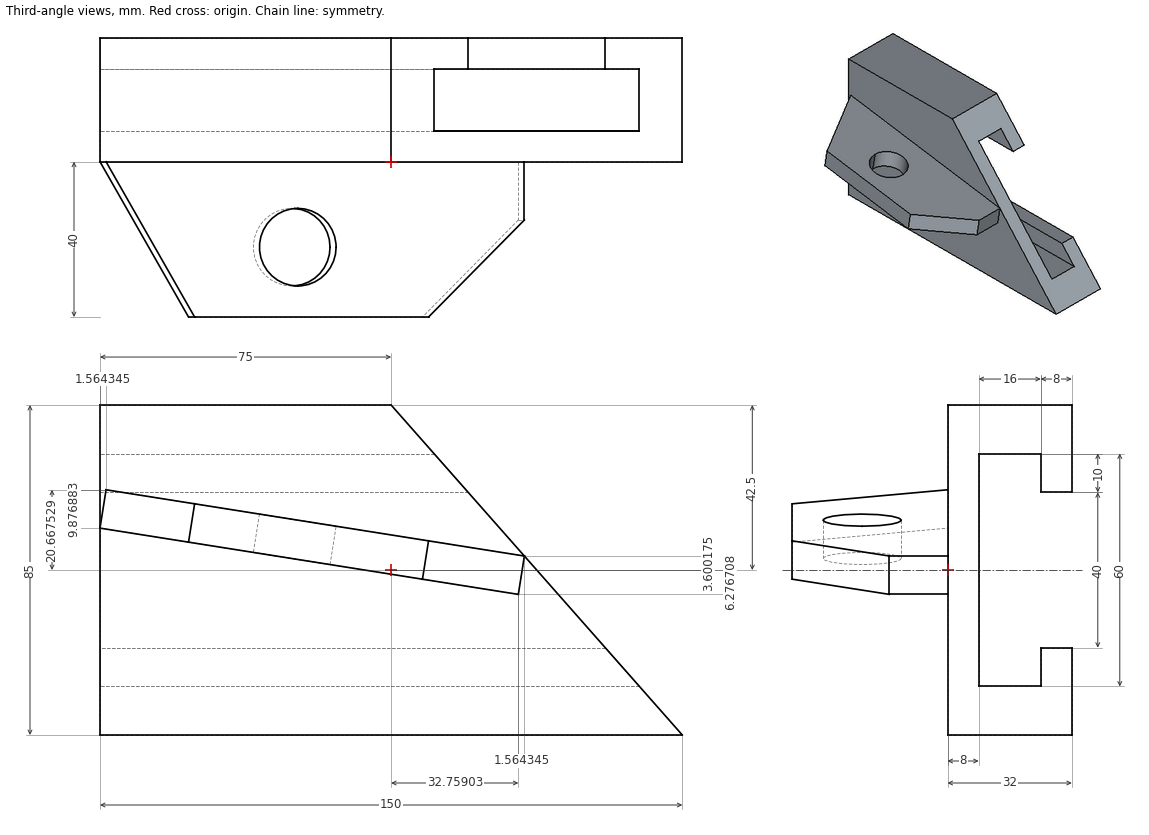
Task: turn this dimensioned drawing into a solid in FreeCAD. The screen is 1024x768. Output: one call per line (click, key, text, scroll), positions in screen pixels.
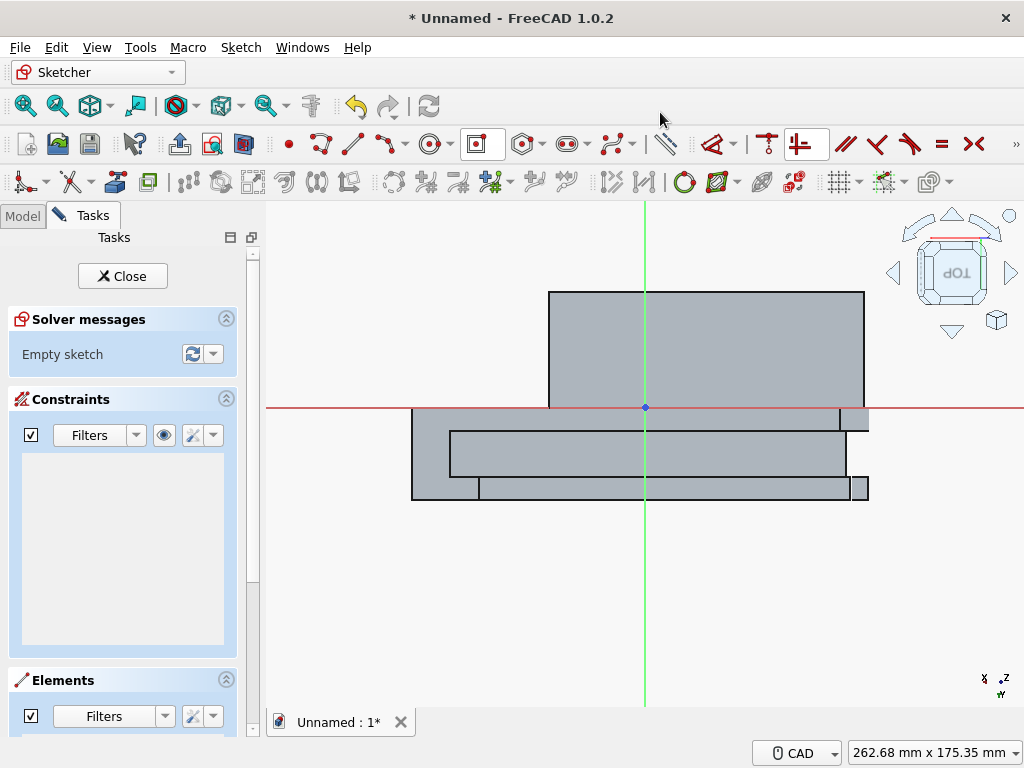
scroll(294, 679, down, 1)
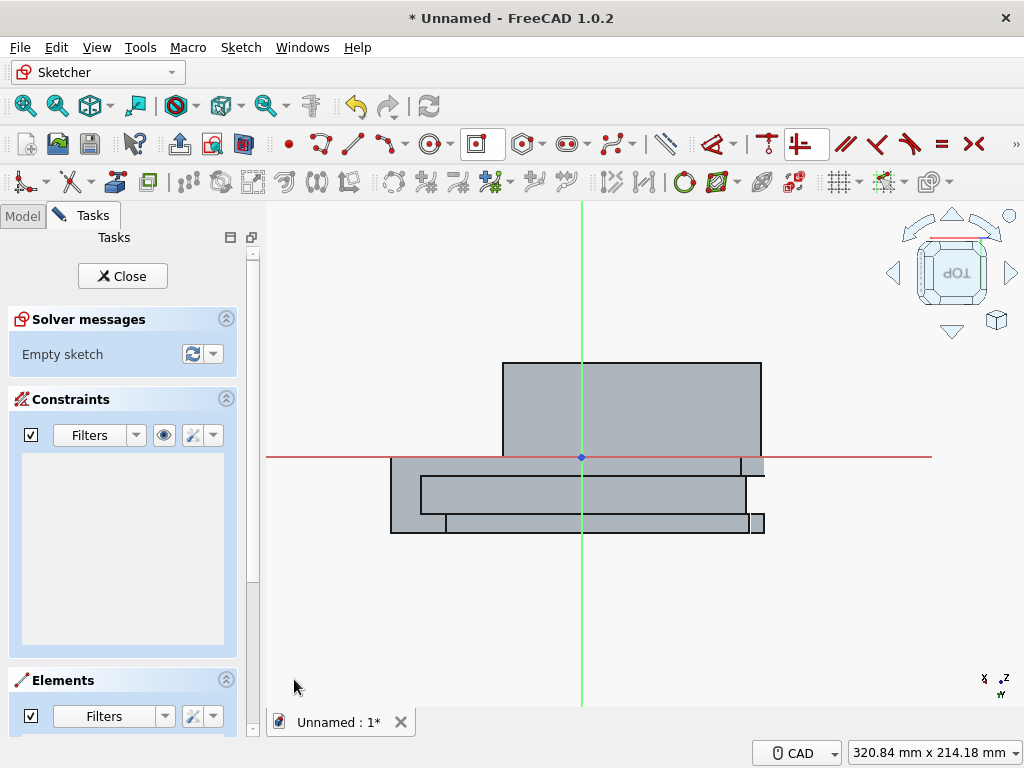
scroll(744, 320, up, 2)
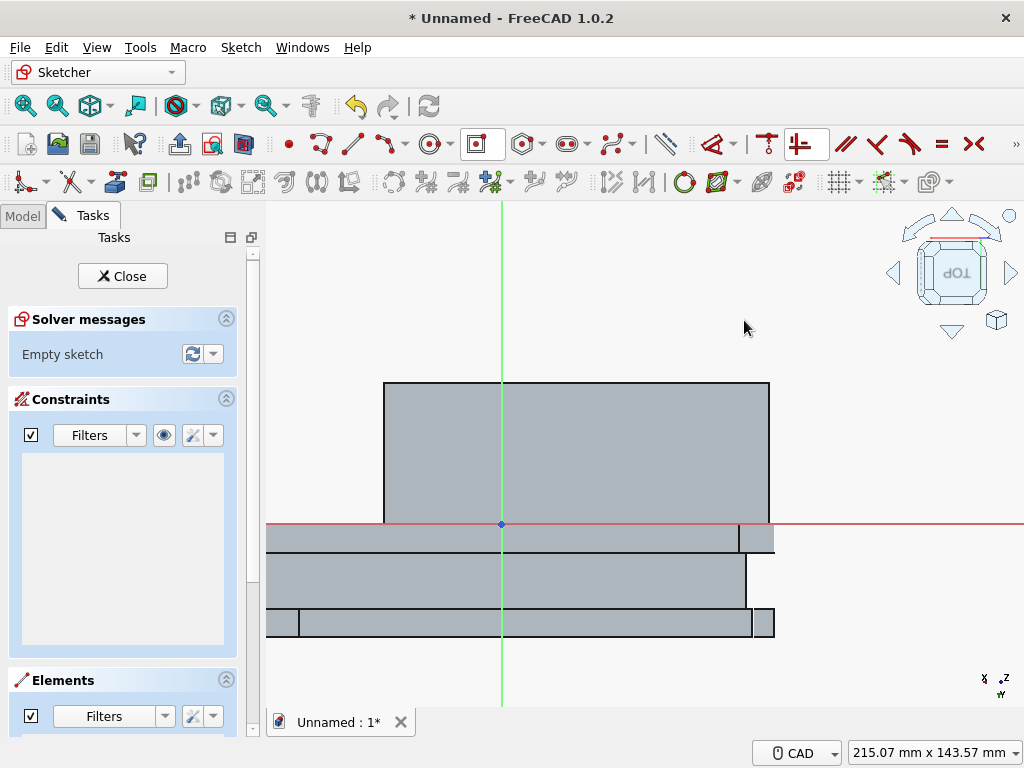
click(322, 144)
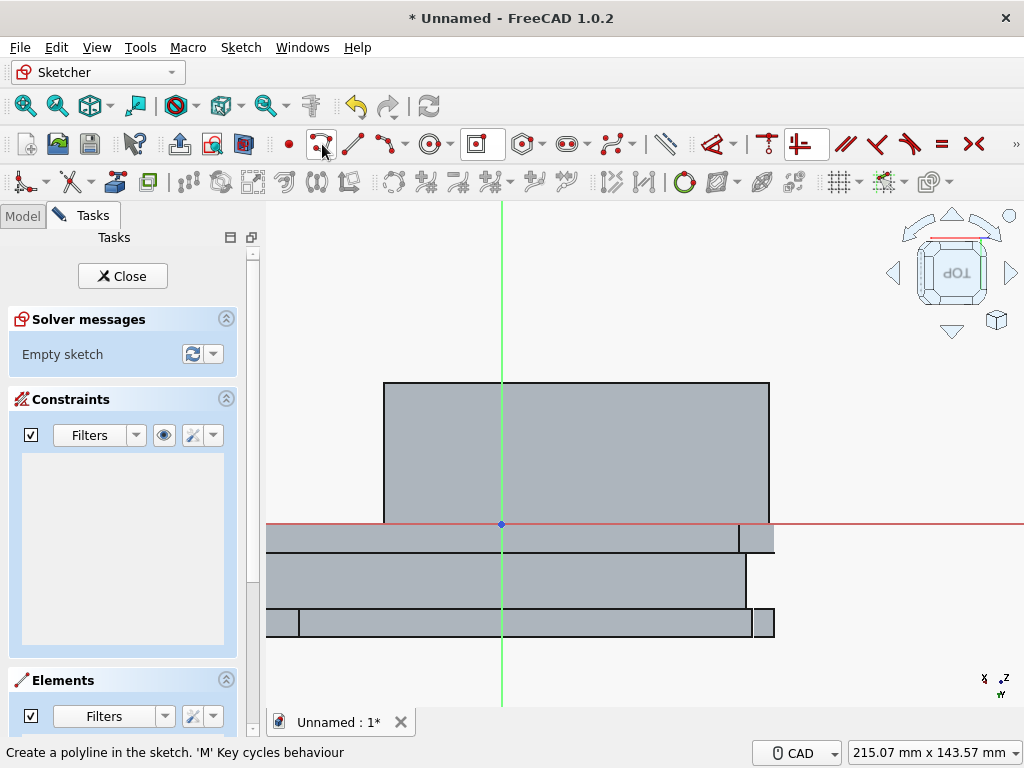
click(384, 471)
click(472, 383)
click(384, 383)
click(384, 472)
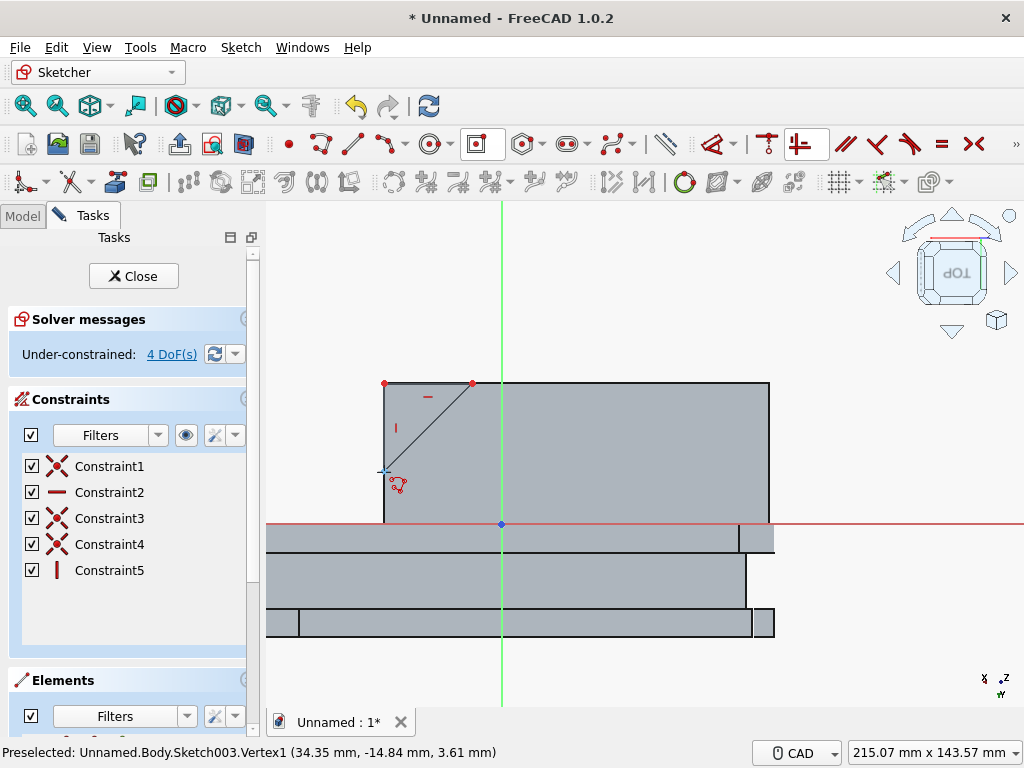
click(687, 383)
click(769, 524)
click(769, 383)
click(687, 384)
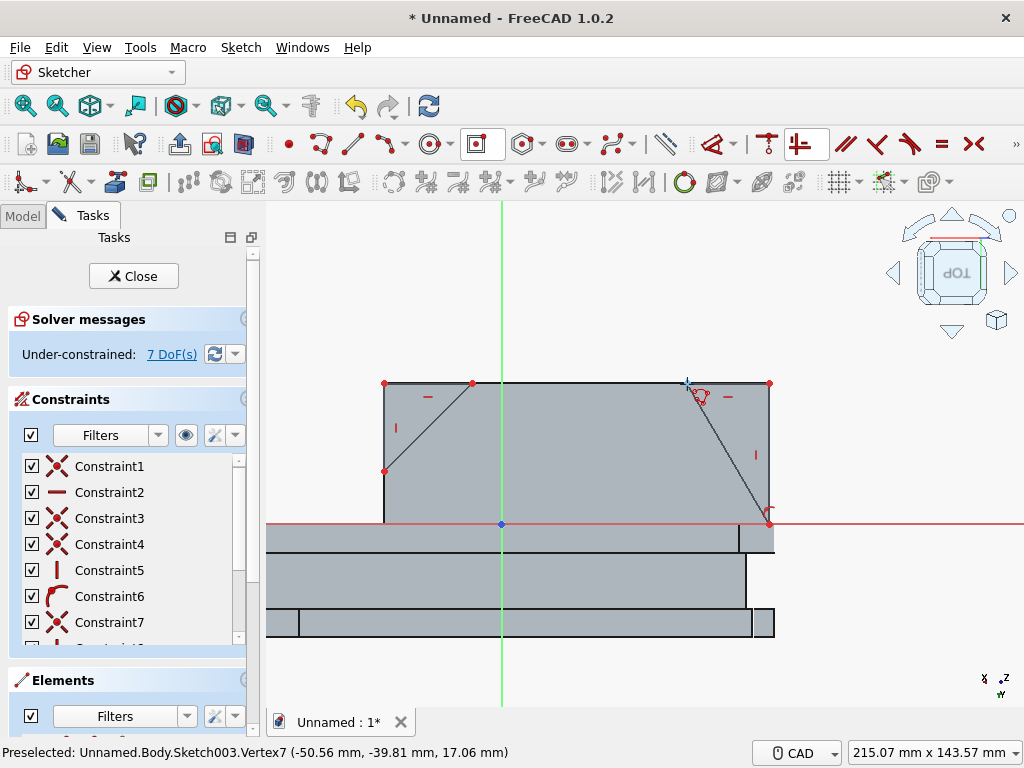
click(430, 144)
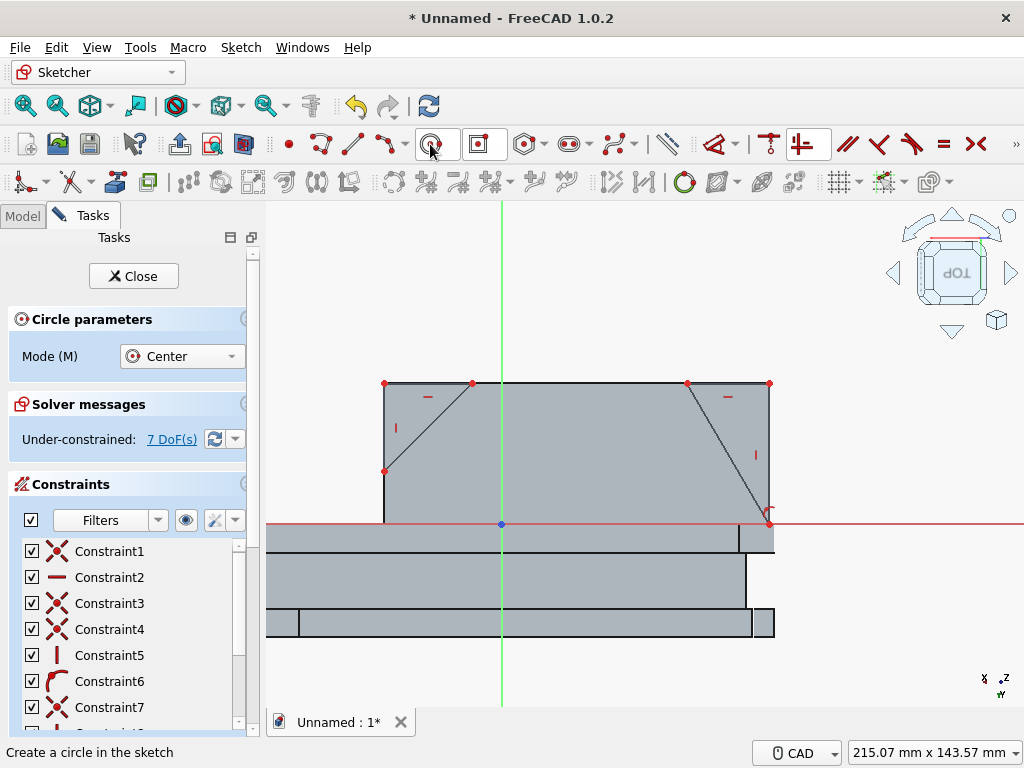
click(592, 447)
move(617, 422)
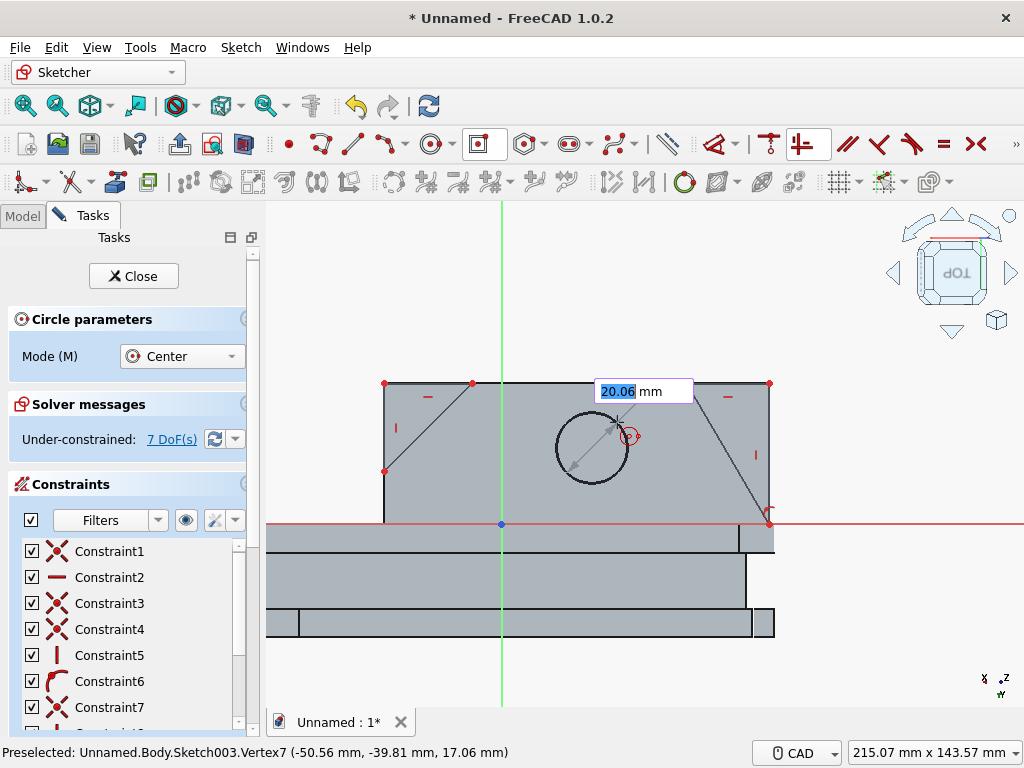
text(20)
key(Return)
key(Escape)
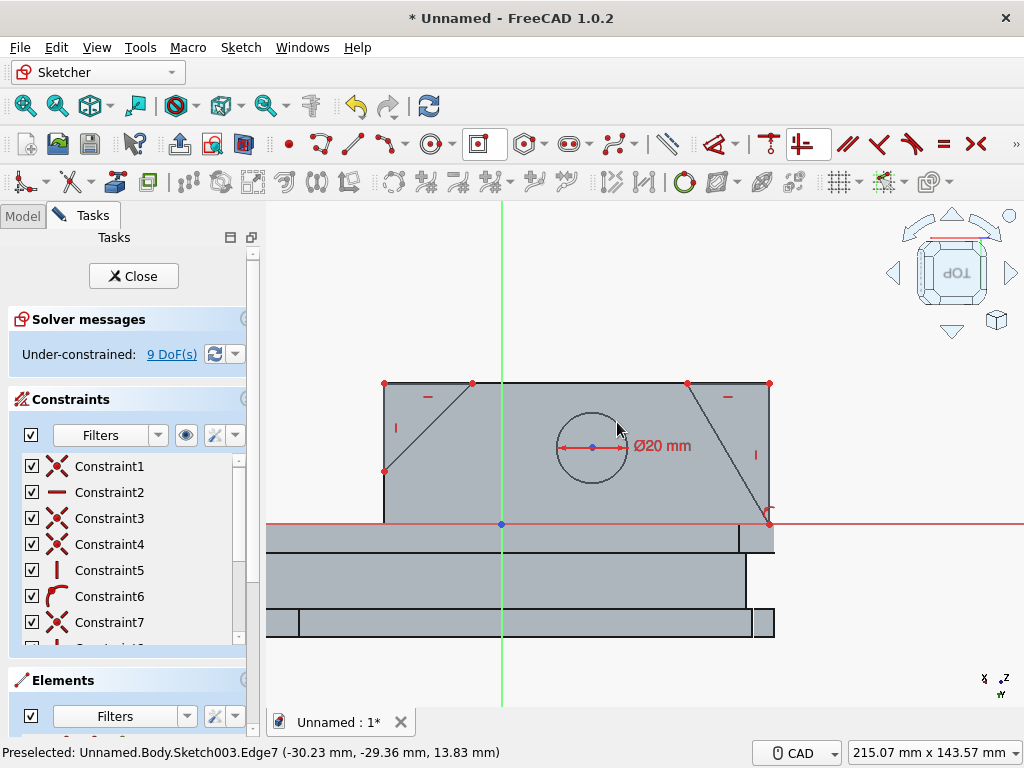
key(d)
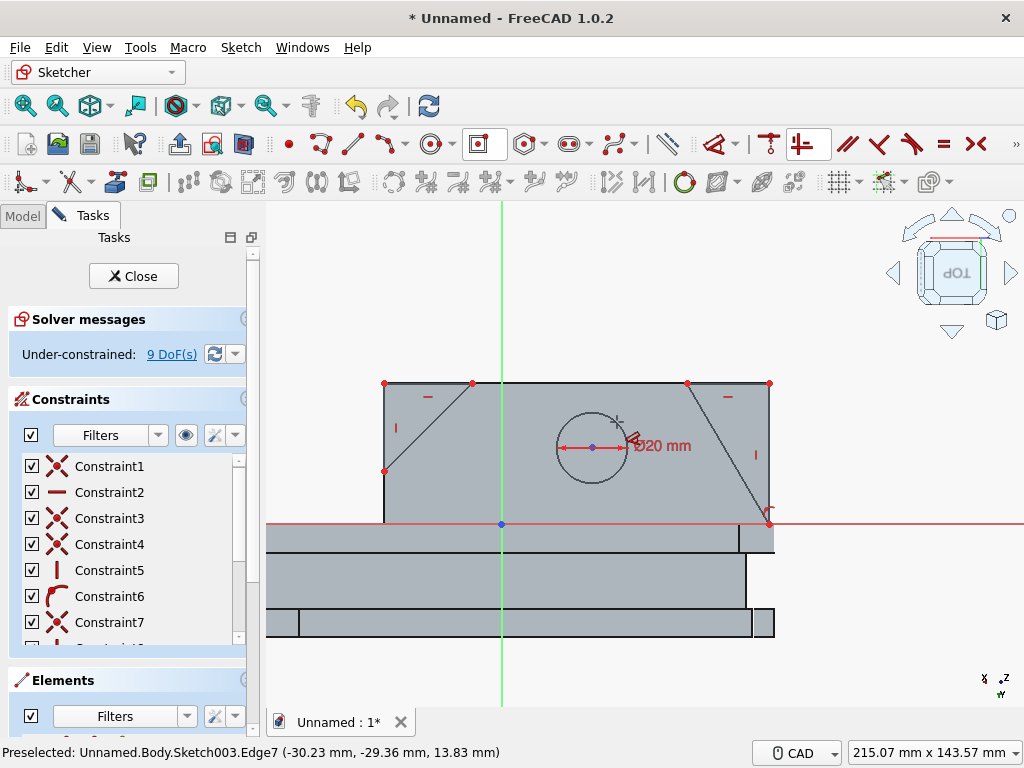
click(446, 384)
click(428, 350)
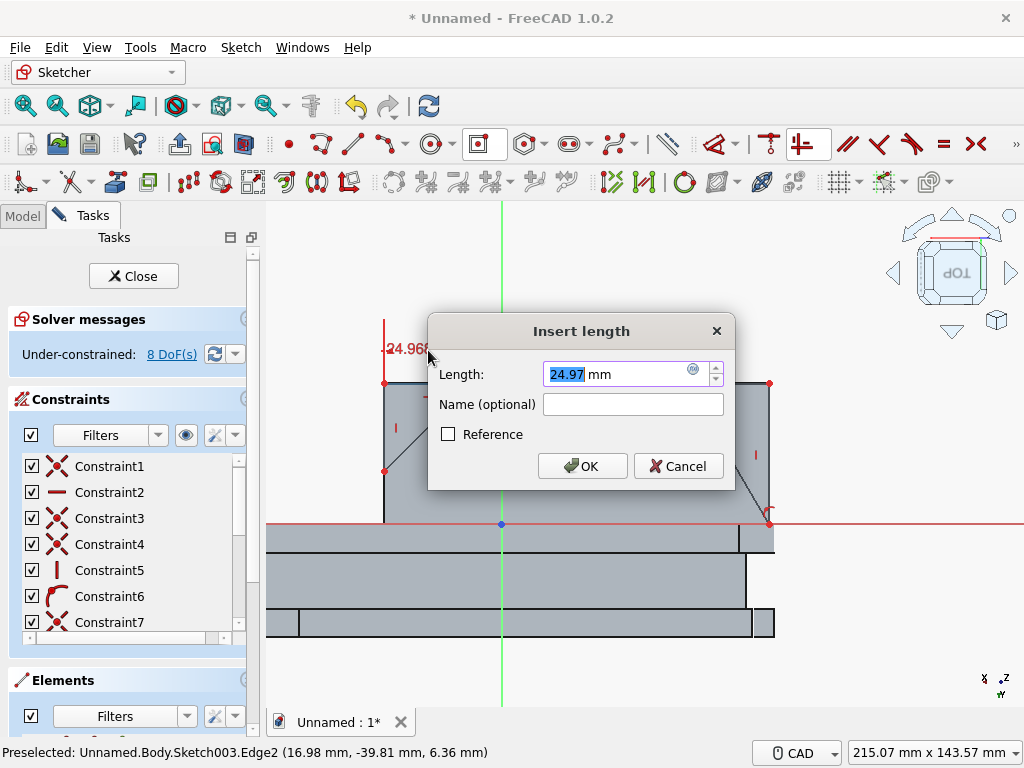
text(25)
key(Return)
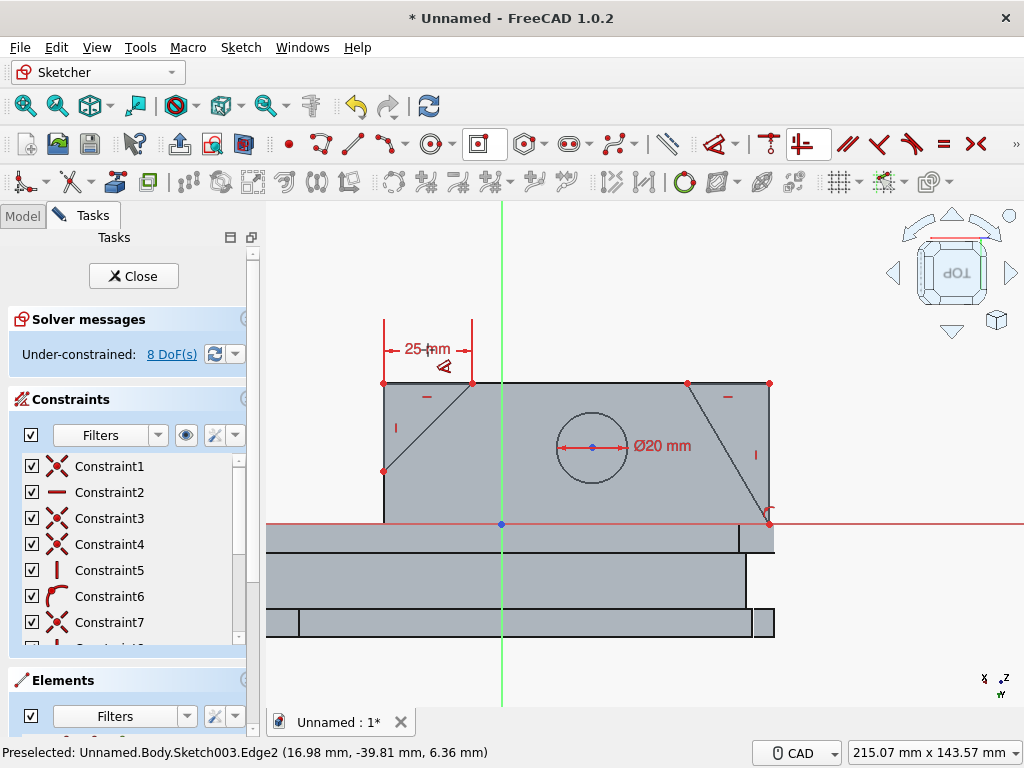
click(384, 410)
click(350, 428)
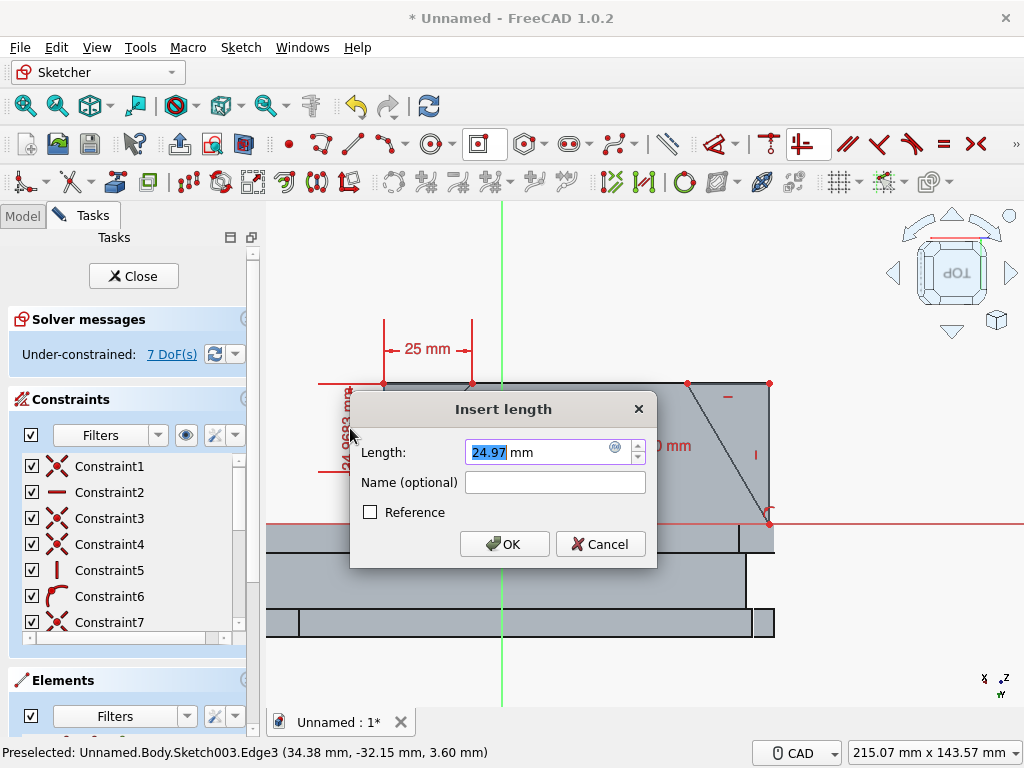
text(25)
key(Return)